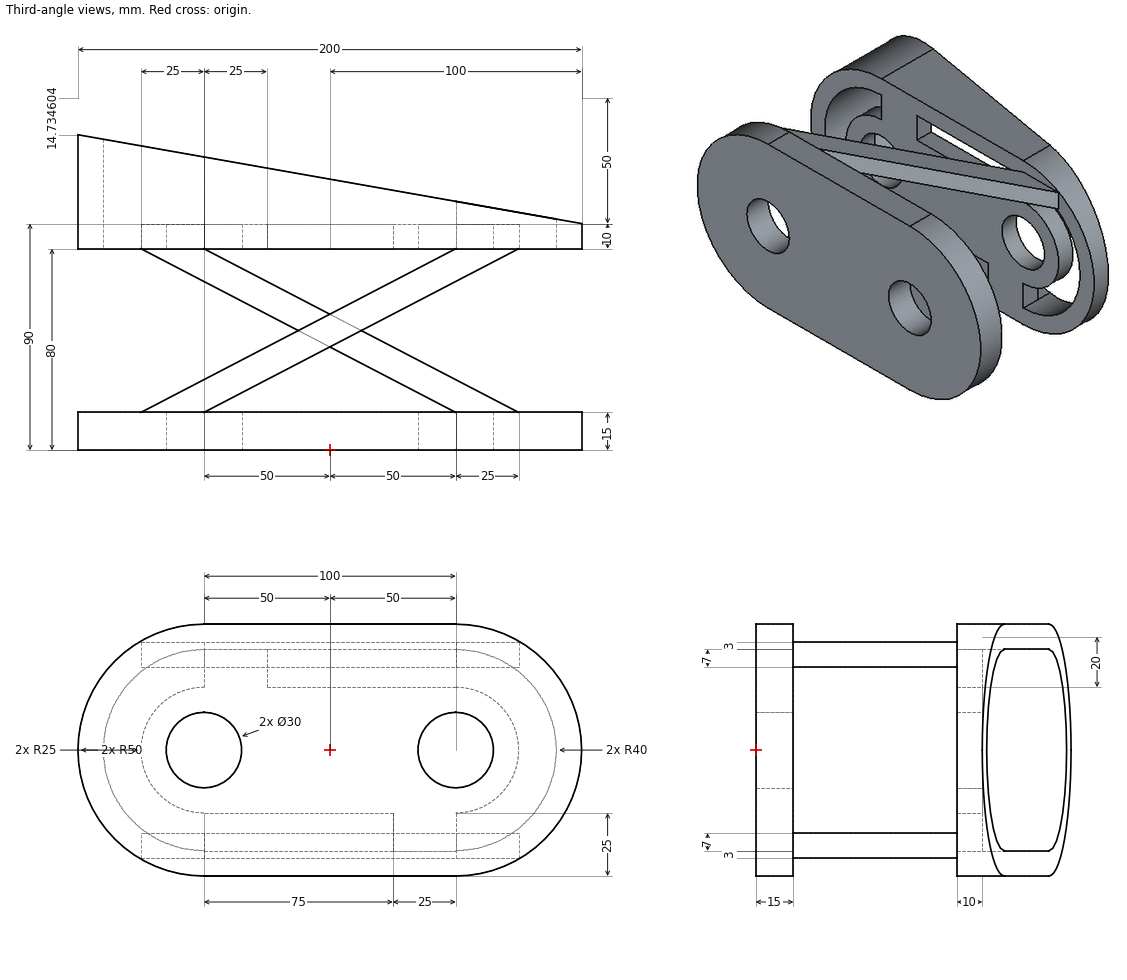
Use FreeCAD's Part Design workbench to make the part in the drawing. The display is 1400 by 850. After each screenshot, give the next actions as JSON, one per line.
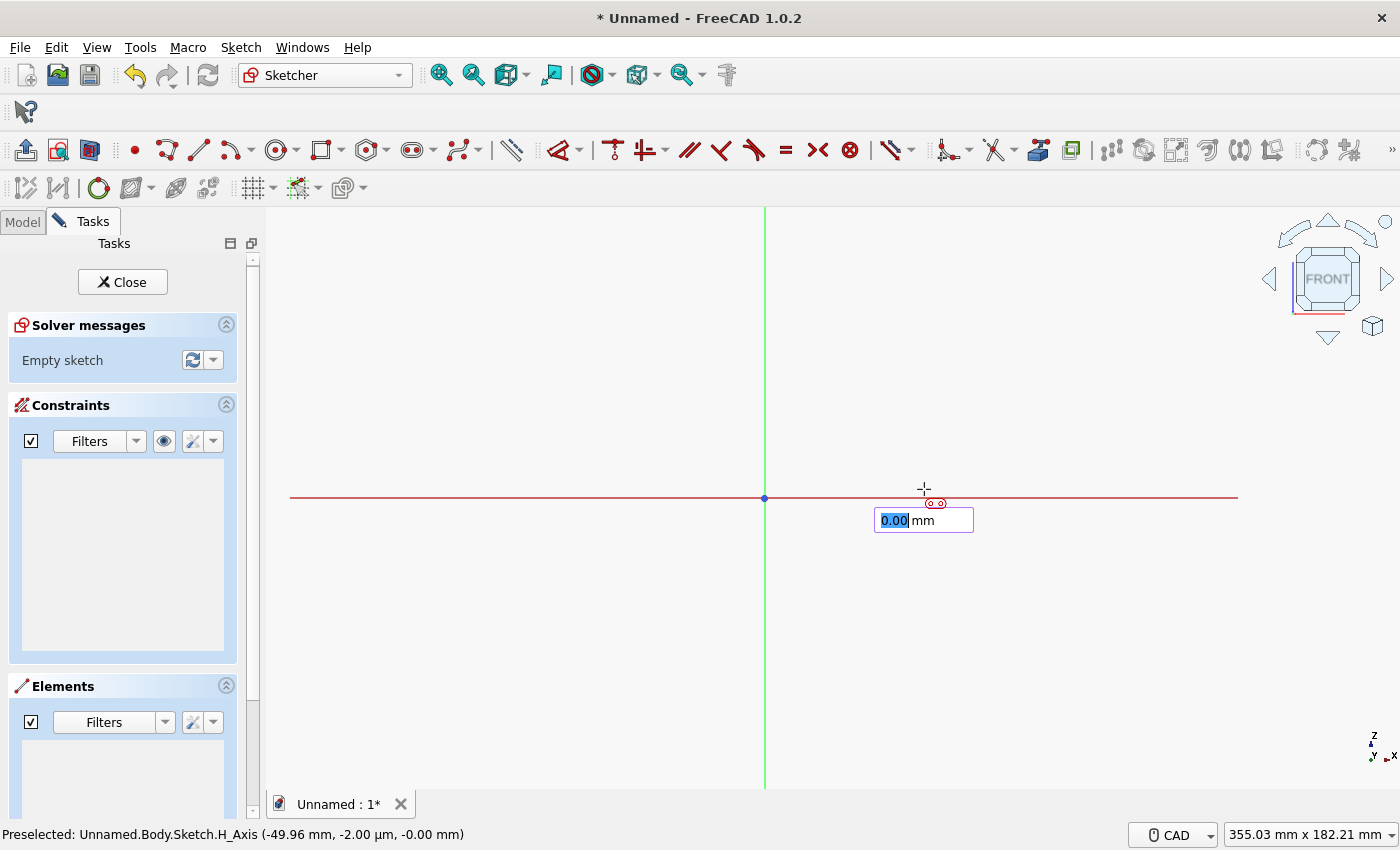
{"action": "left_click", "coordinate": [812, 658]}
{"action": "key", "text": "Escape"}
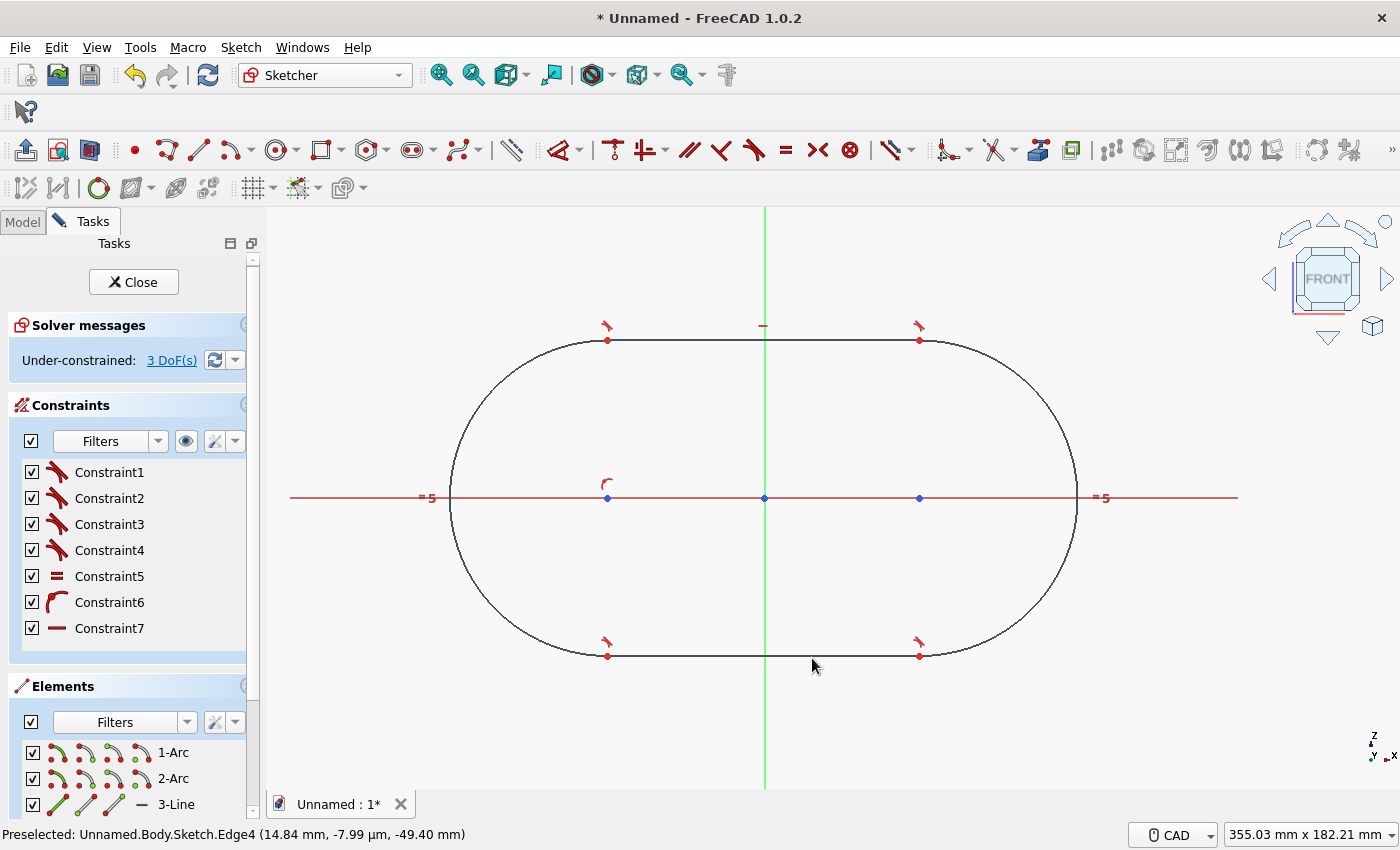
{"action": "left_click", "coordinate": [558, 150]}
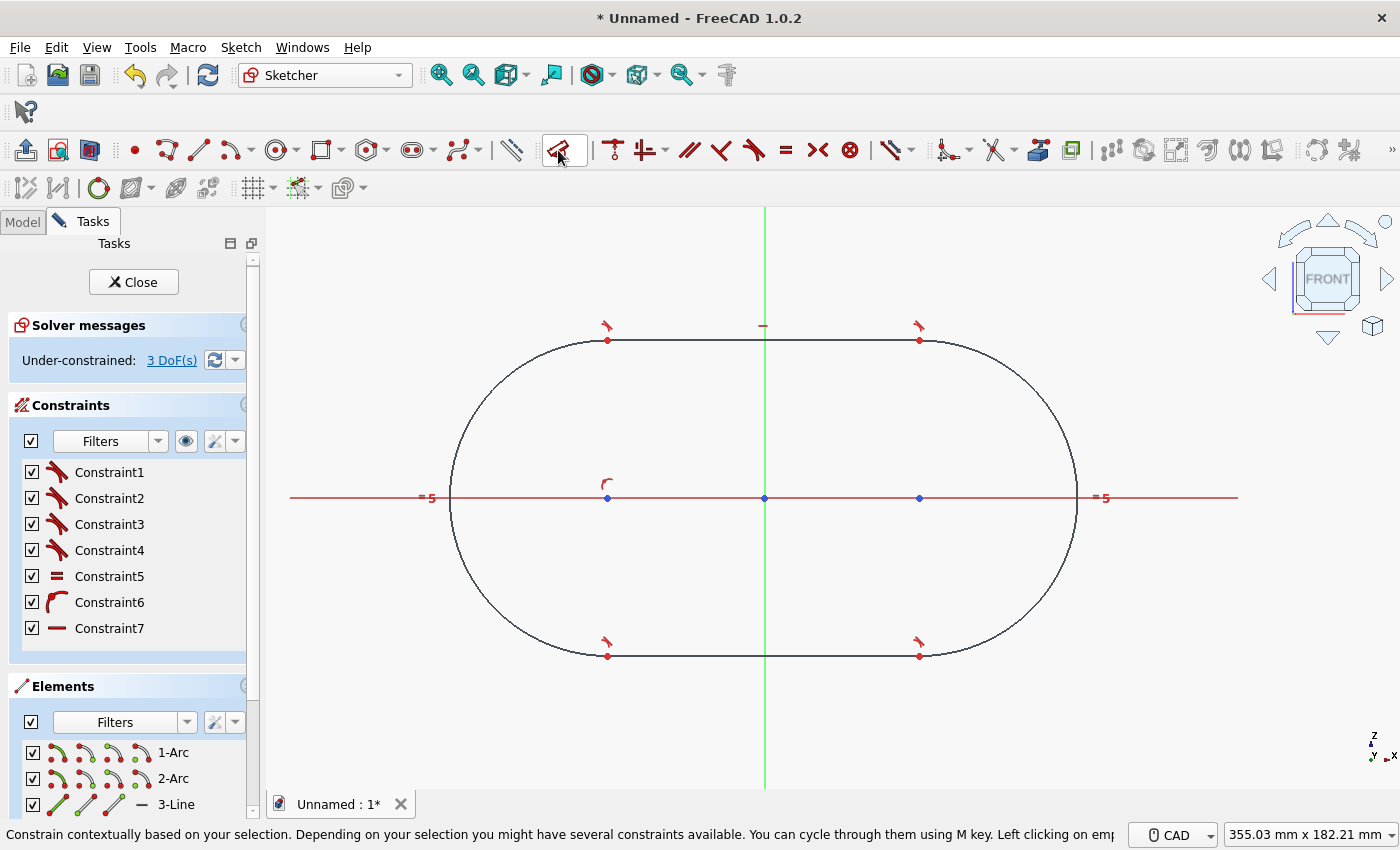
{"action": "left_click", "coordinate": [480, 405]}
{"action": "left_click", "coordinate": [454, 386]}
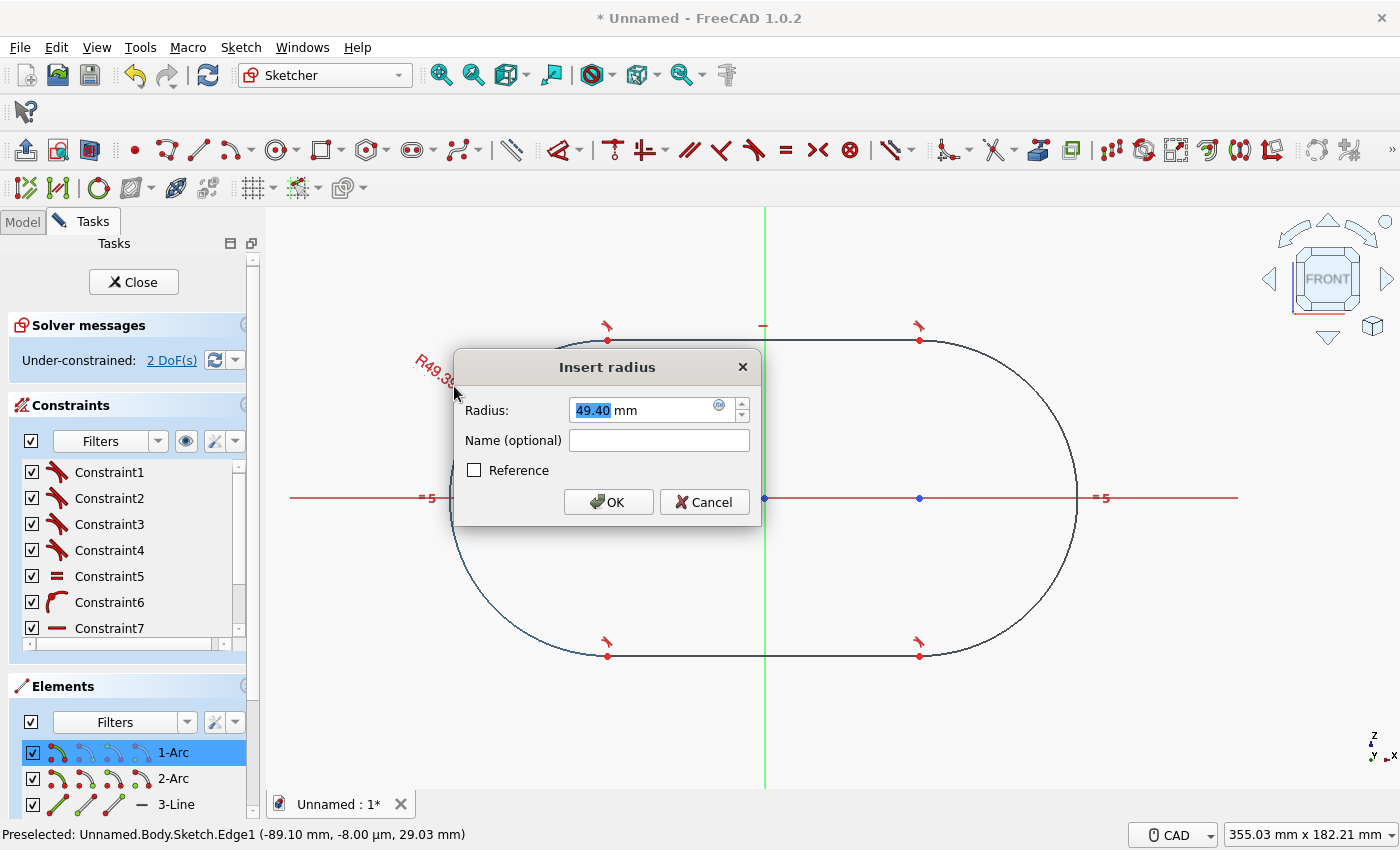
{"action": "type", "text": "50"}
{"action": "key", "text": "Return"}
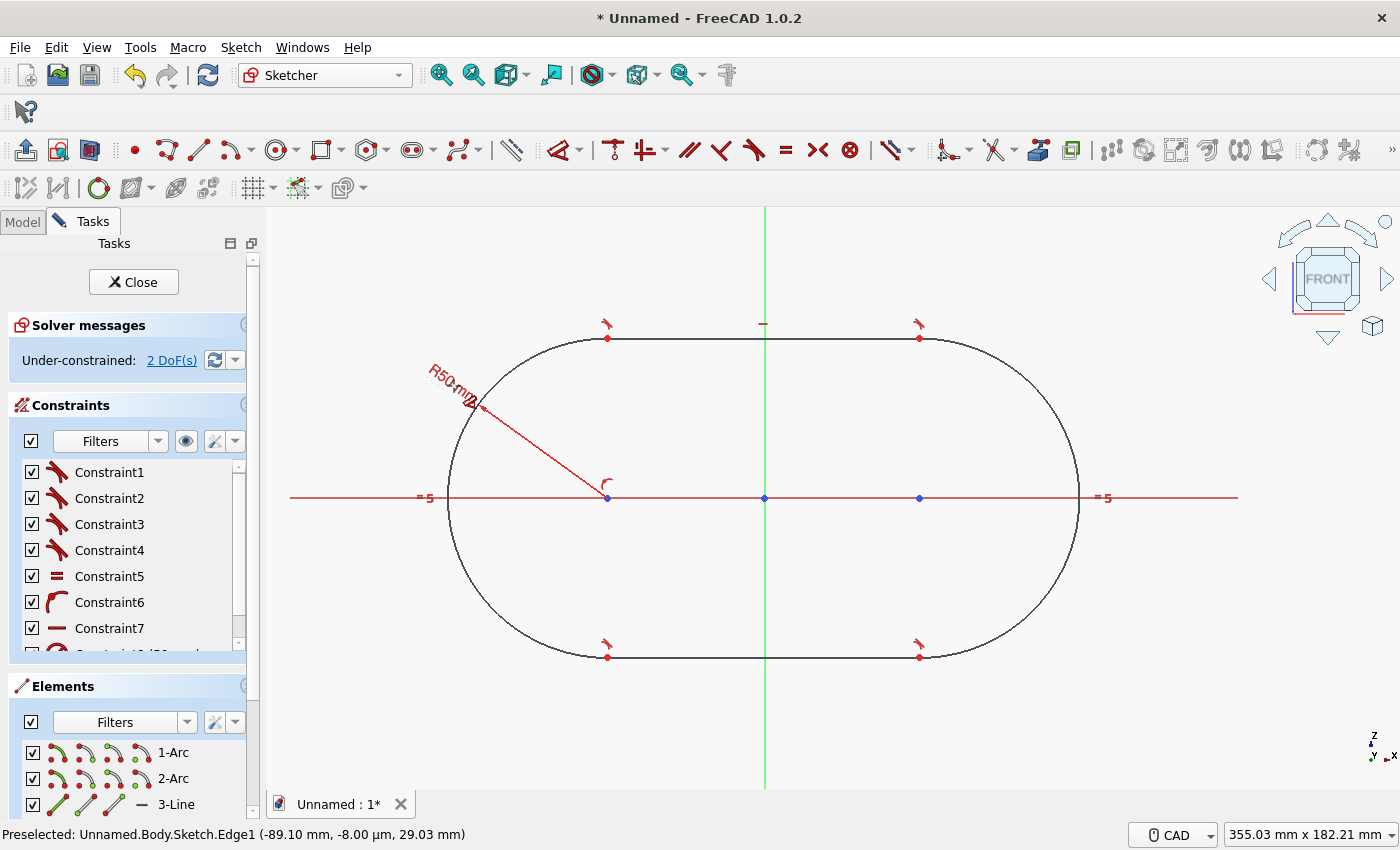
{"action": "left_click", "coordinate": [701, 339]}
{"action": "left_click", "coordinate": [692, 305]}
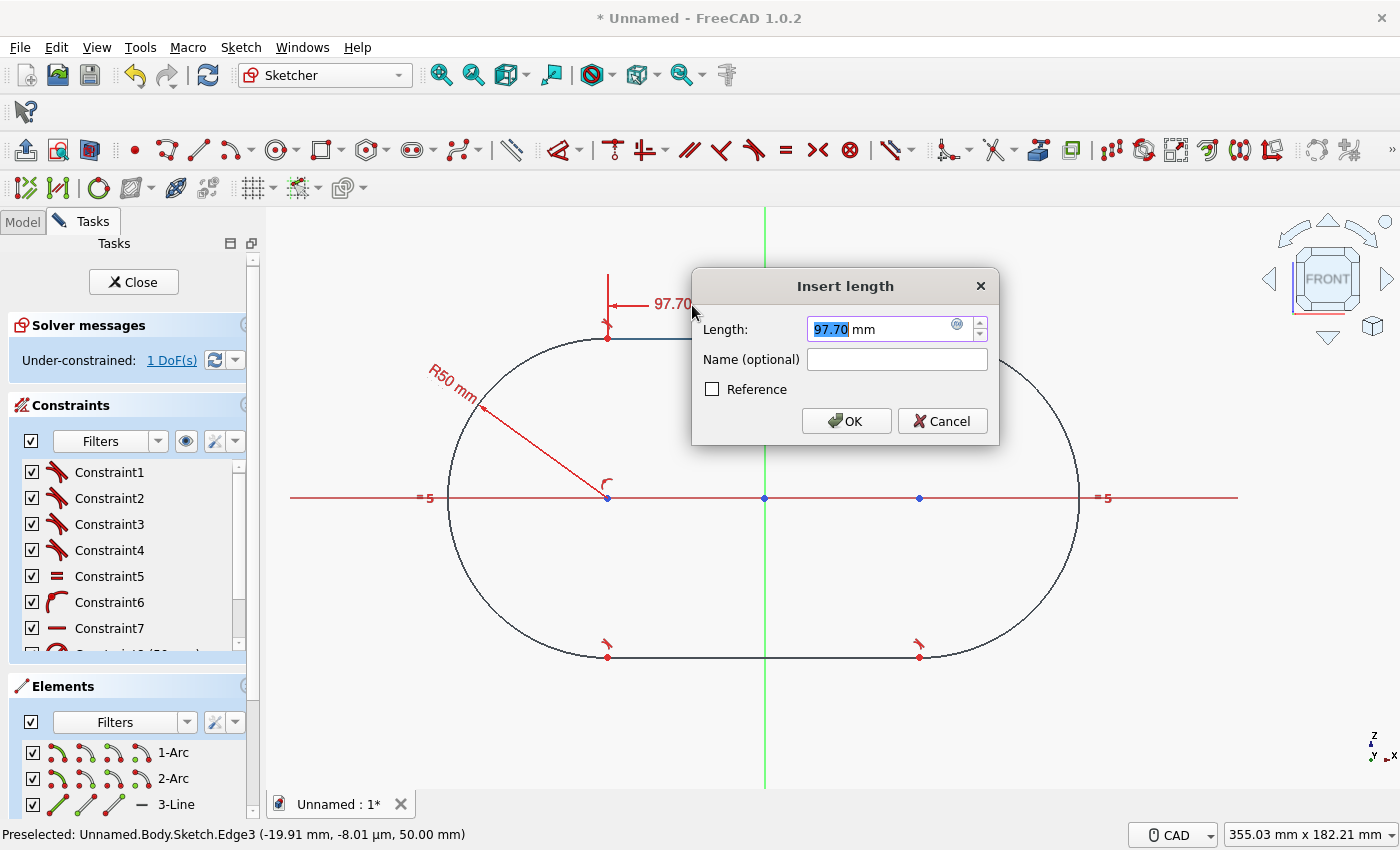
{"action": "type", "text": "100"}
{"action": "key", "text": "Return"}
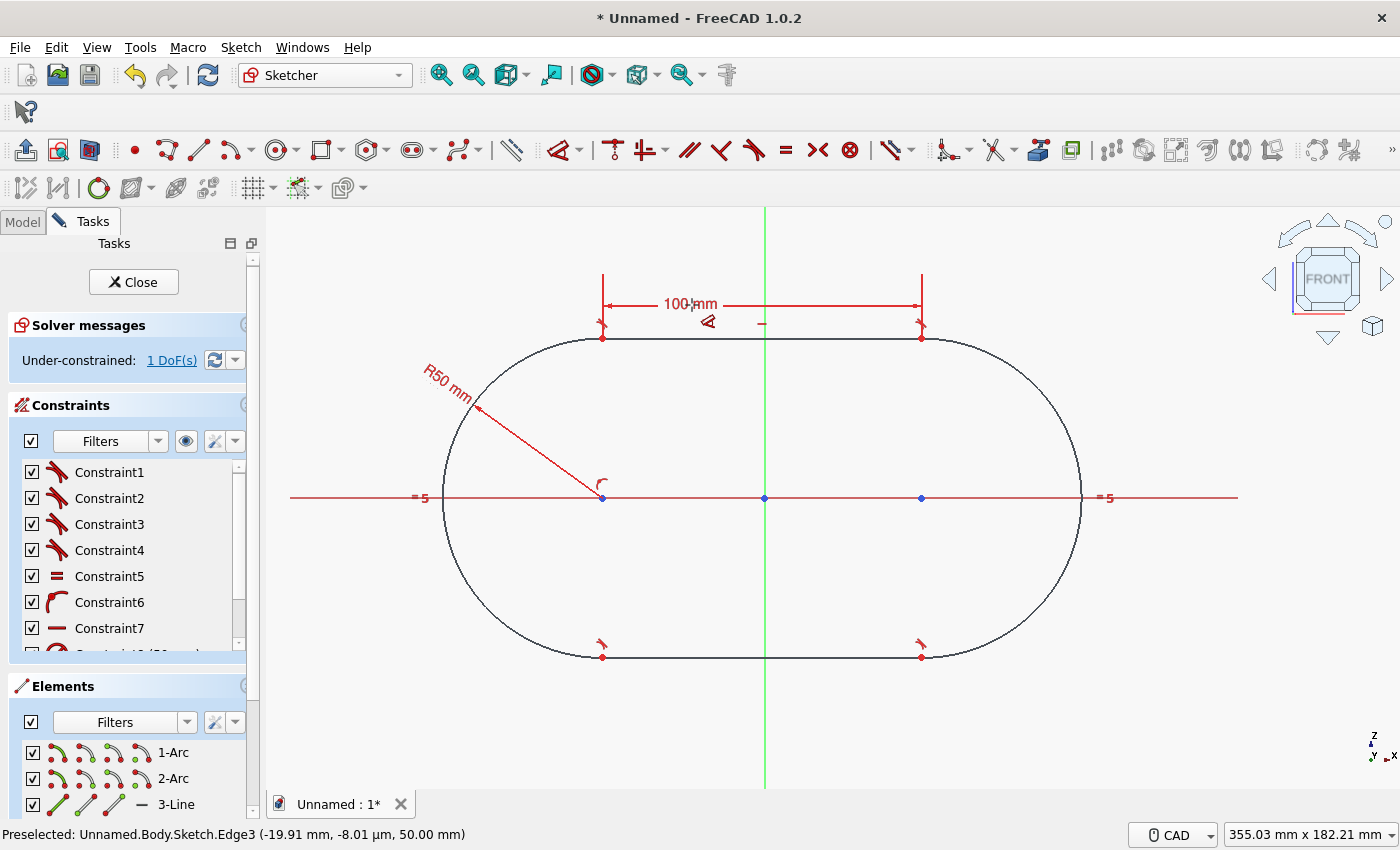
{"action": "left_click", "coordinate": [603, 339]}
{"action": "left_click", "coordinate": [684, 532]}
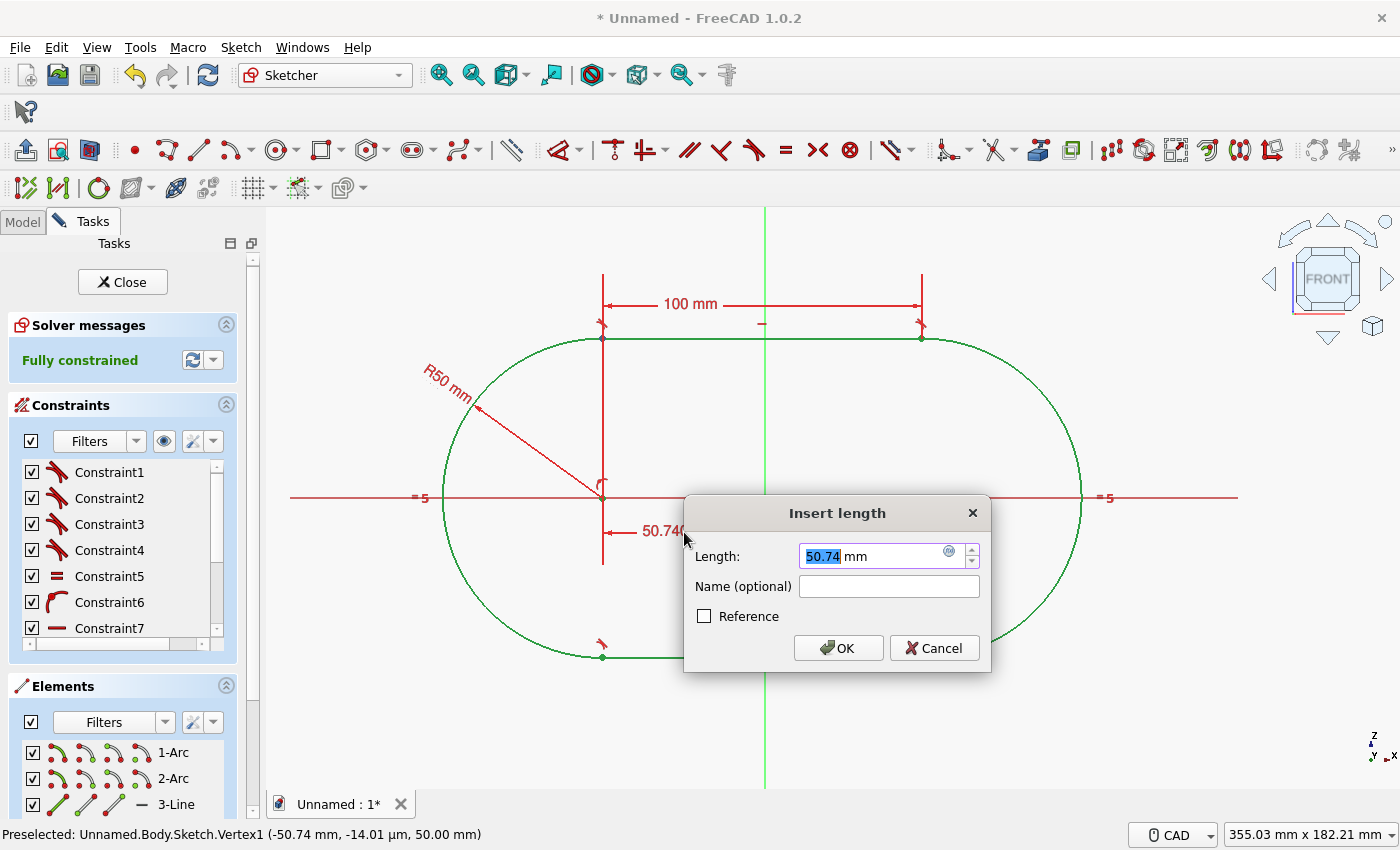
{"action": "type", "text": "50"}
{"action": "key", "text": "Return"}
{"action": "key", "text": "Escape"}